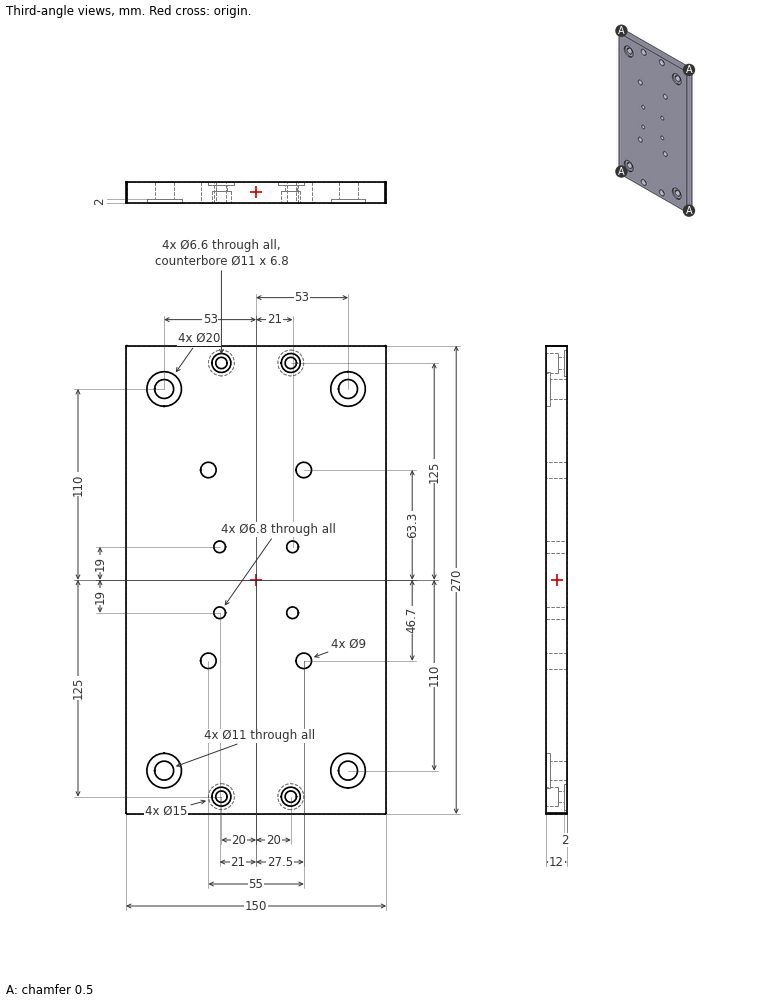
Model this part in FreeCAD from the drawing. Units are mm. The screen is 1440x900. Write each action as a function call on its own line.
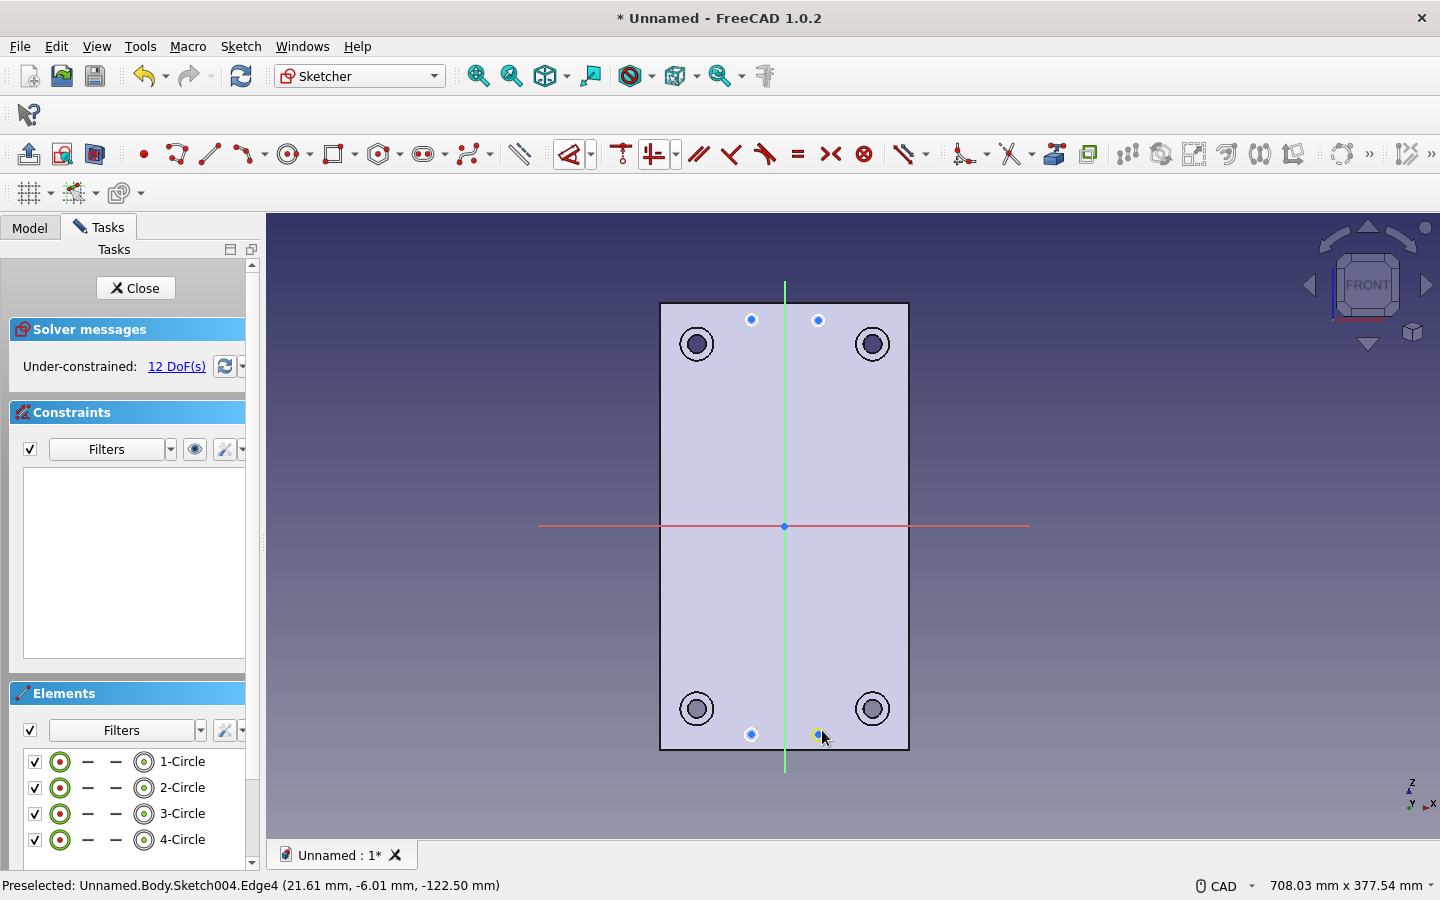
scroll(756, 316, up, 5)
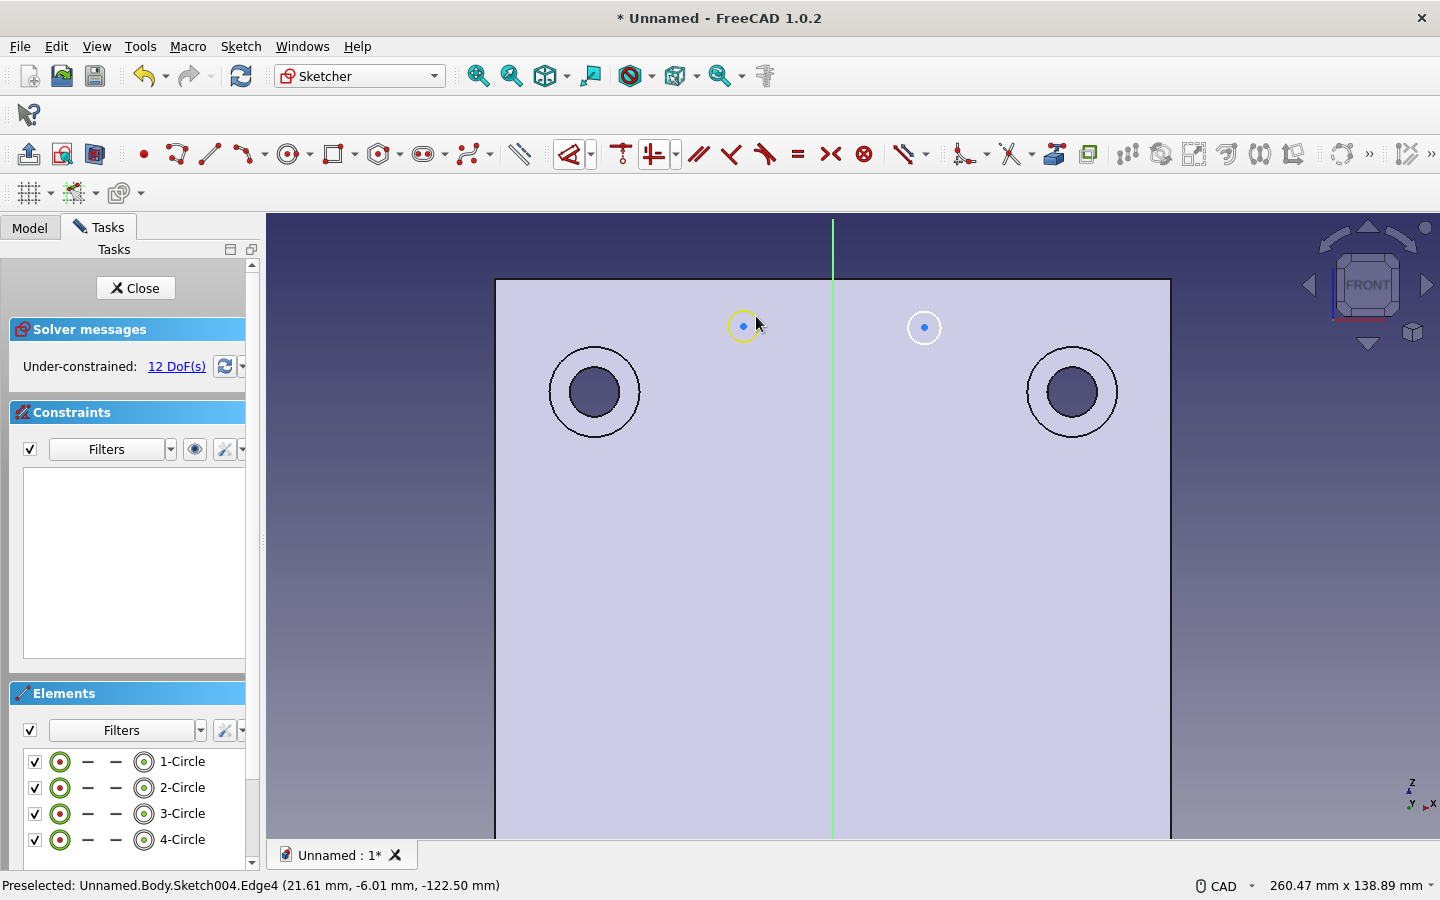
click(755, 315)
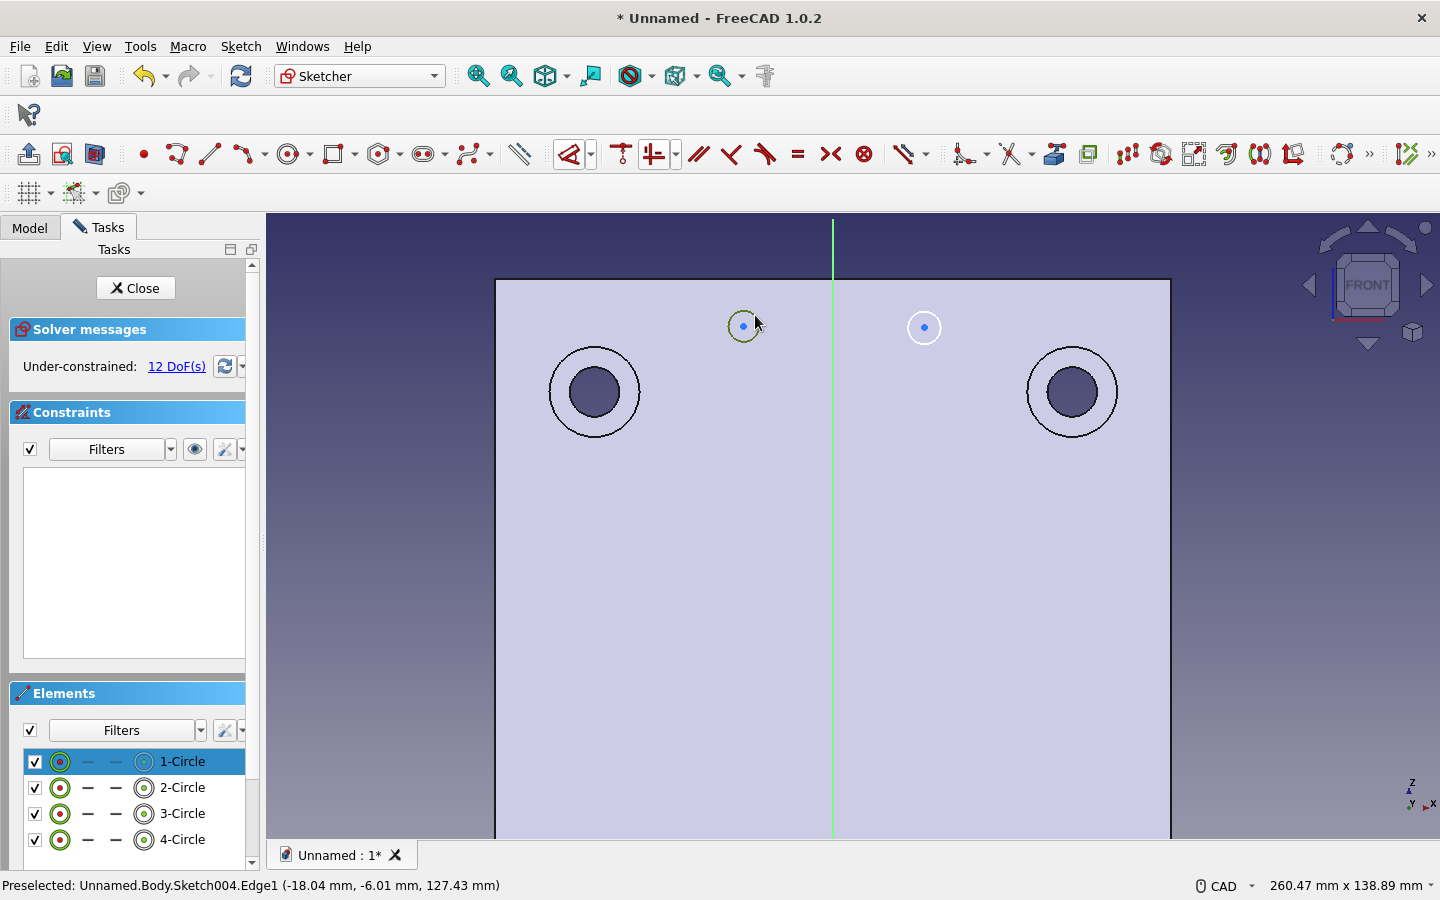
click(936, 316)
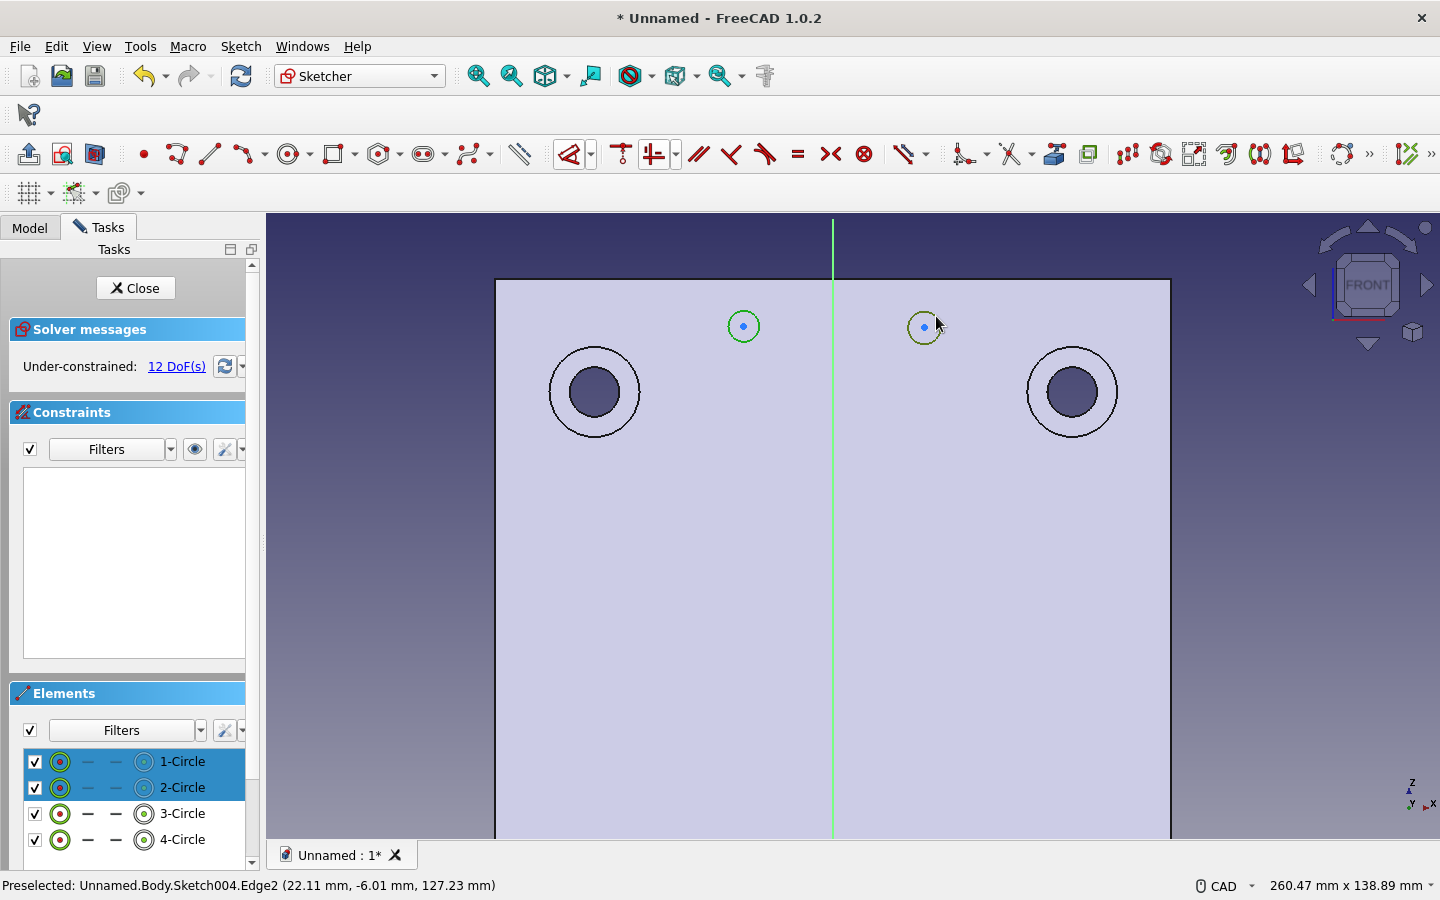
scroll(756, 315, down, 5)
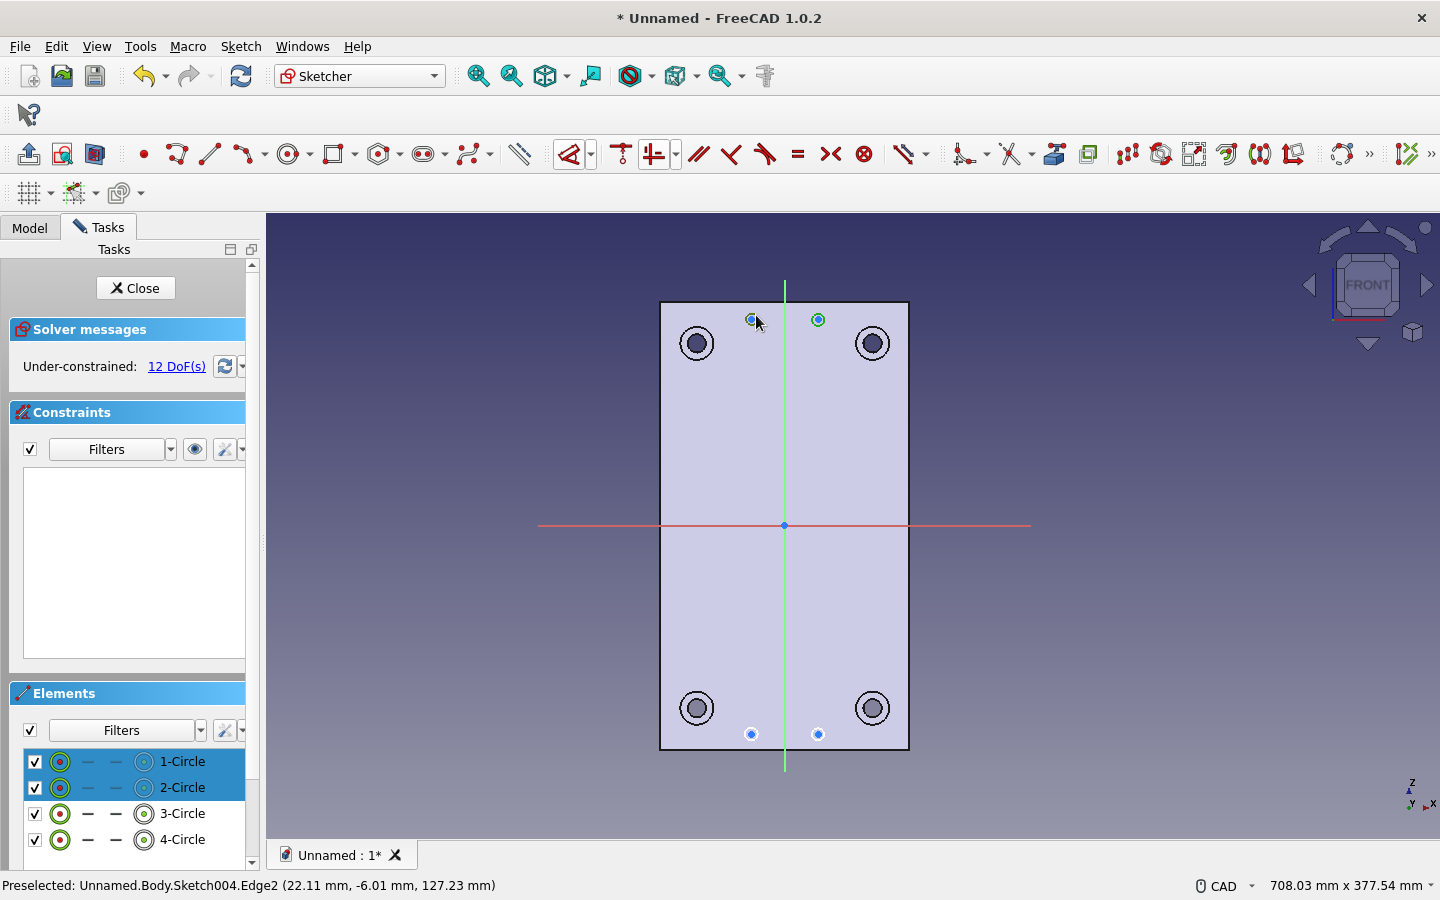
scroll(756, 730, up, 4)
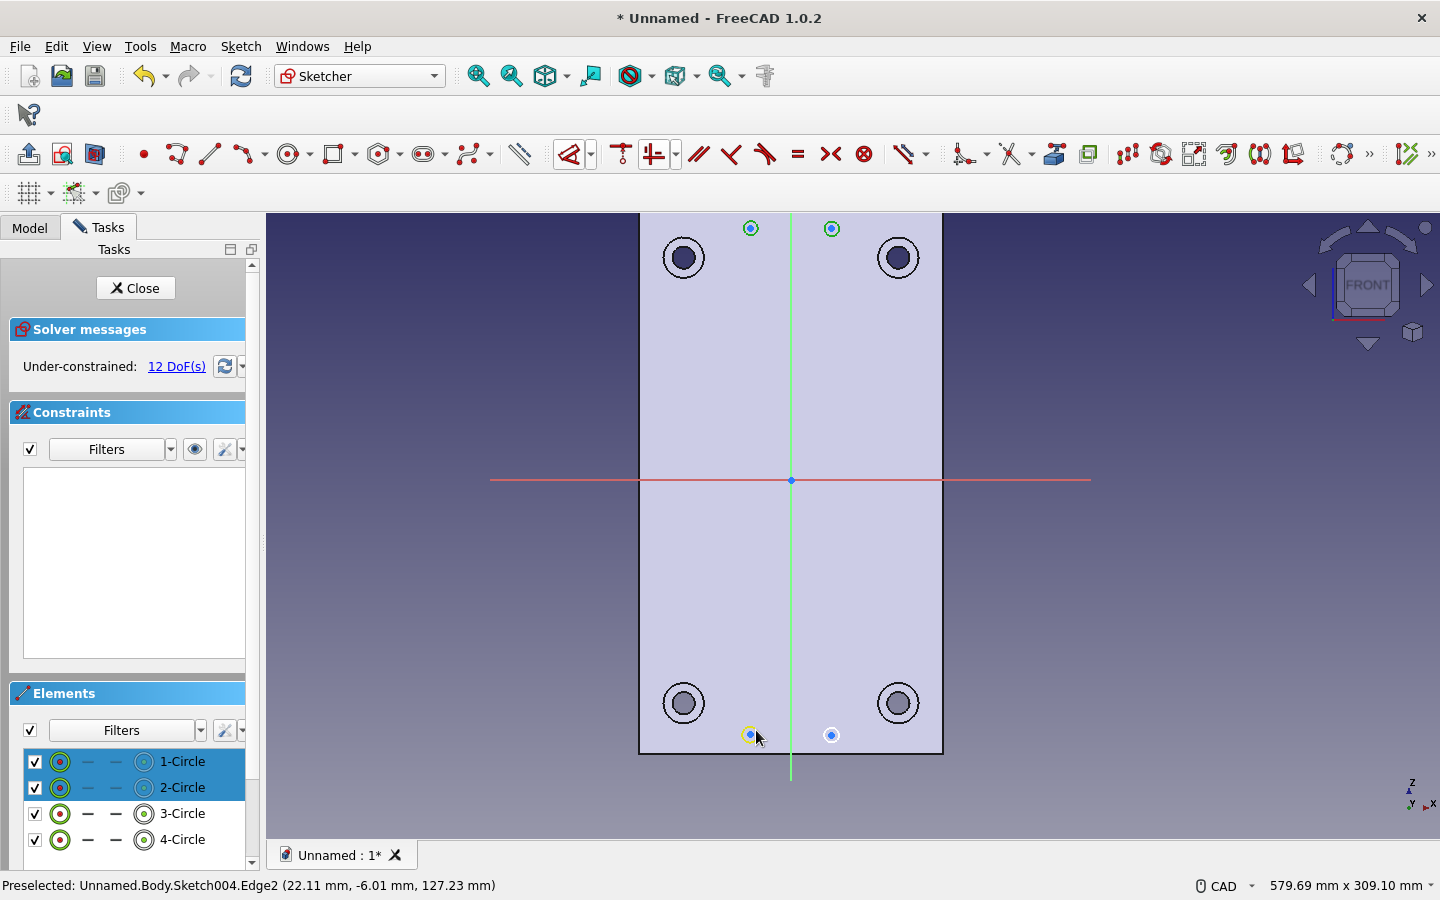
click(755, 728)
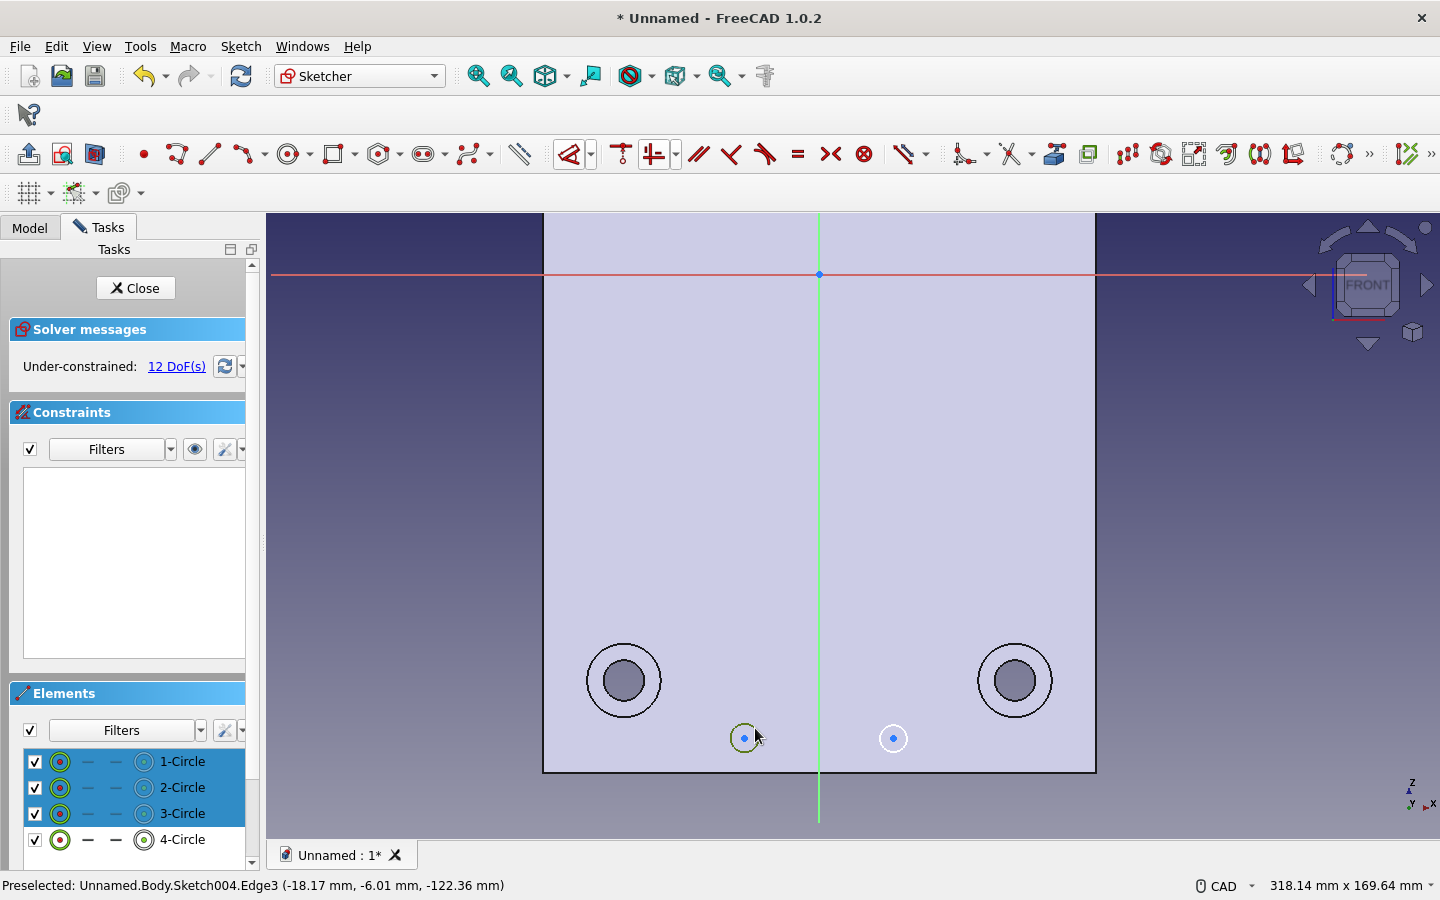
click(903, 729)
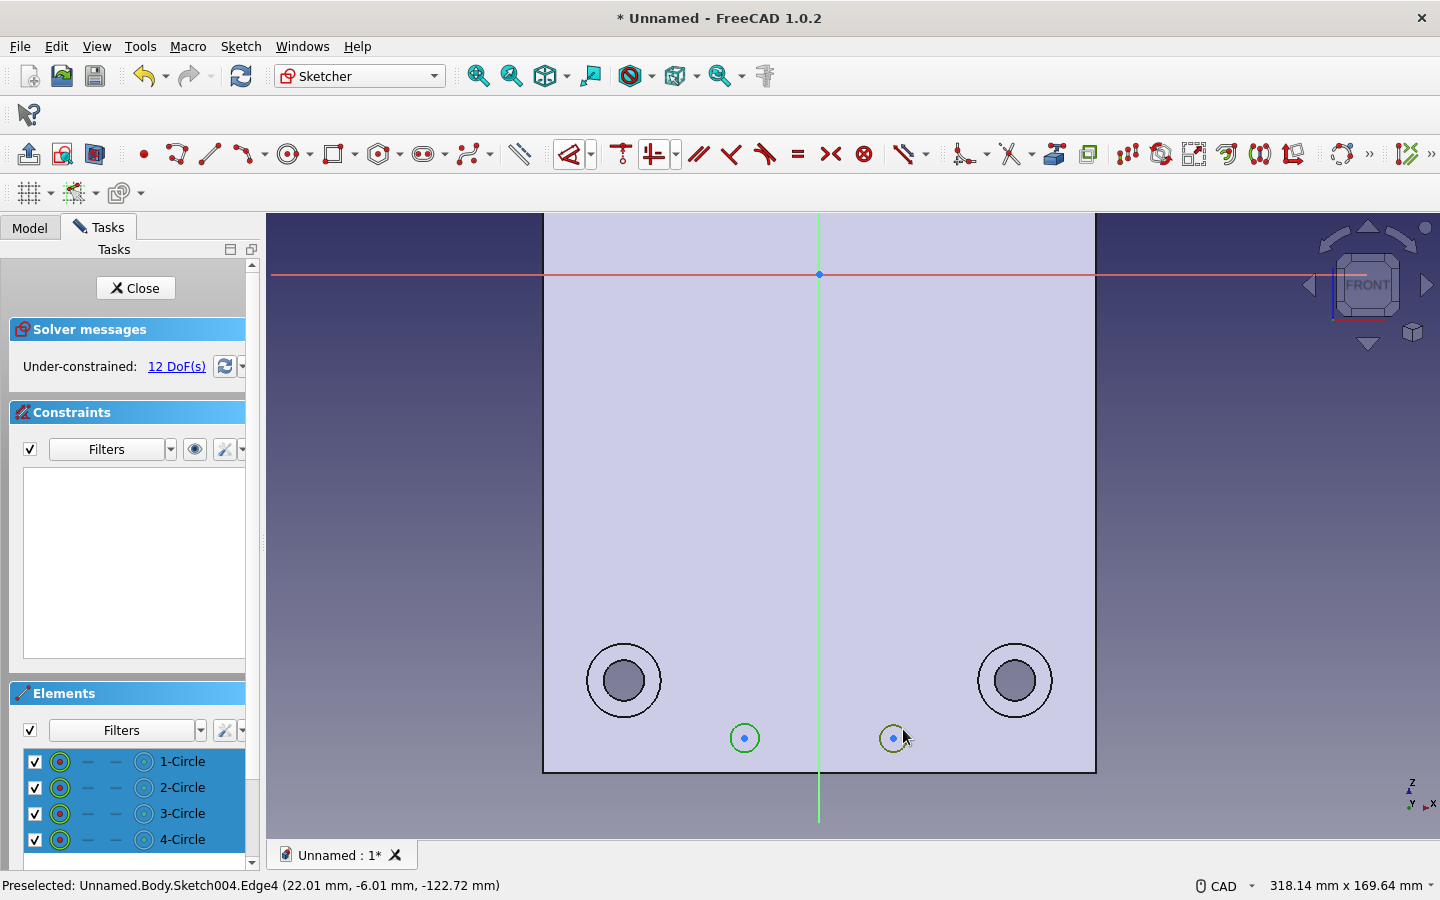
click(798, 154)